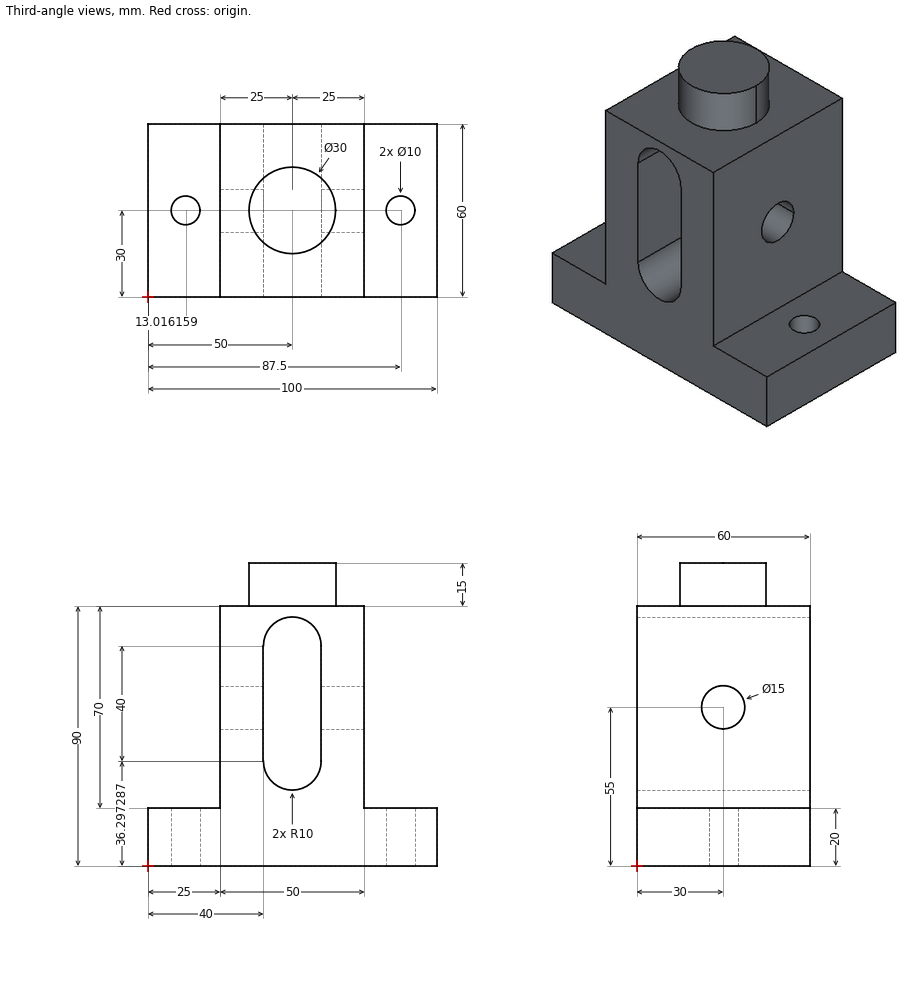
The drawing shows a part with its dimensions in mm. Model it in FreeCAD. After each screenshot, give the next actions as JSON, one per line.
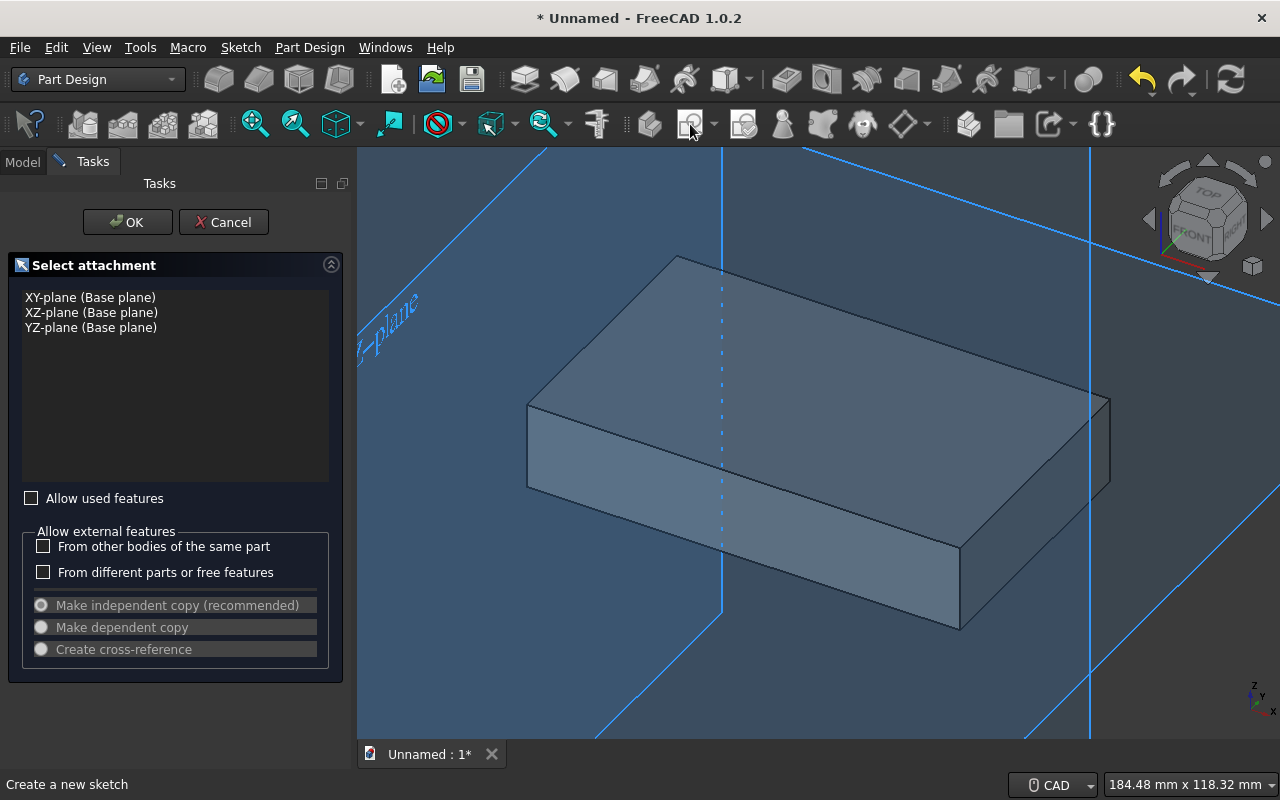
{"action": "left_click", "coordinate": [82, 312]}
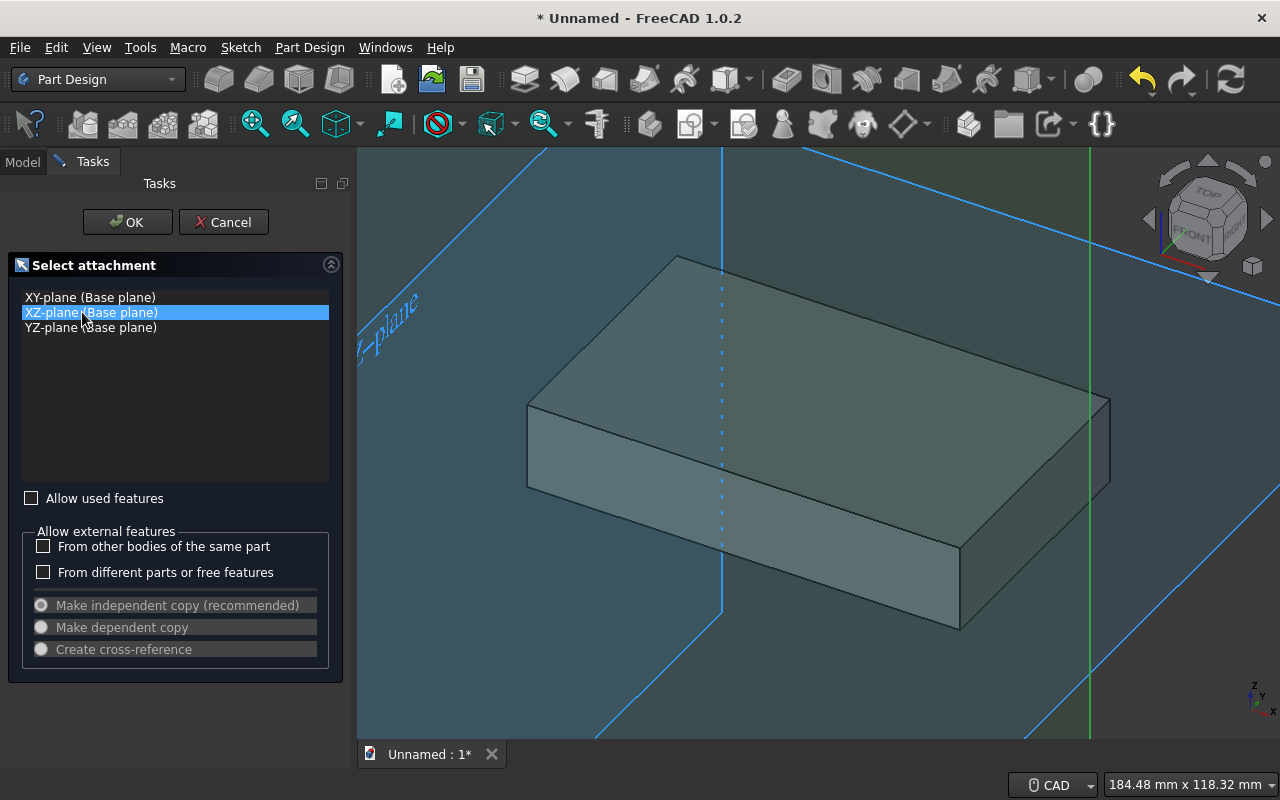
{"action": "left_click", "coordinate": [128, 222]}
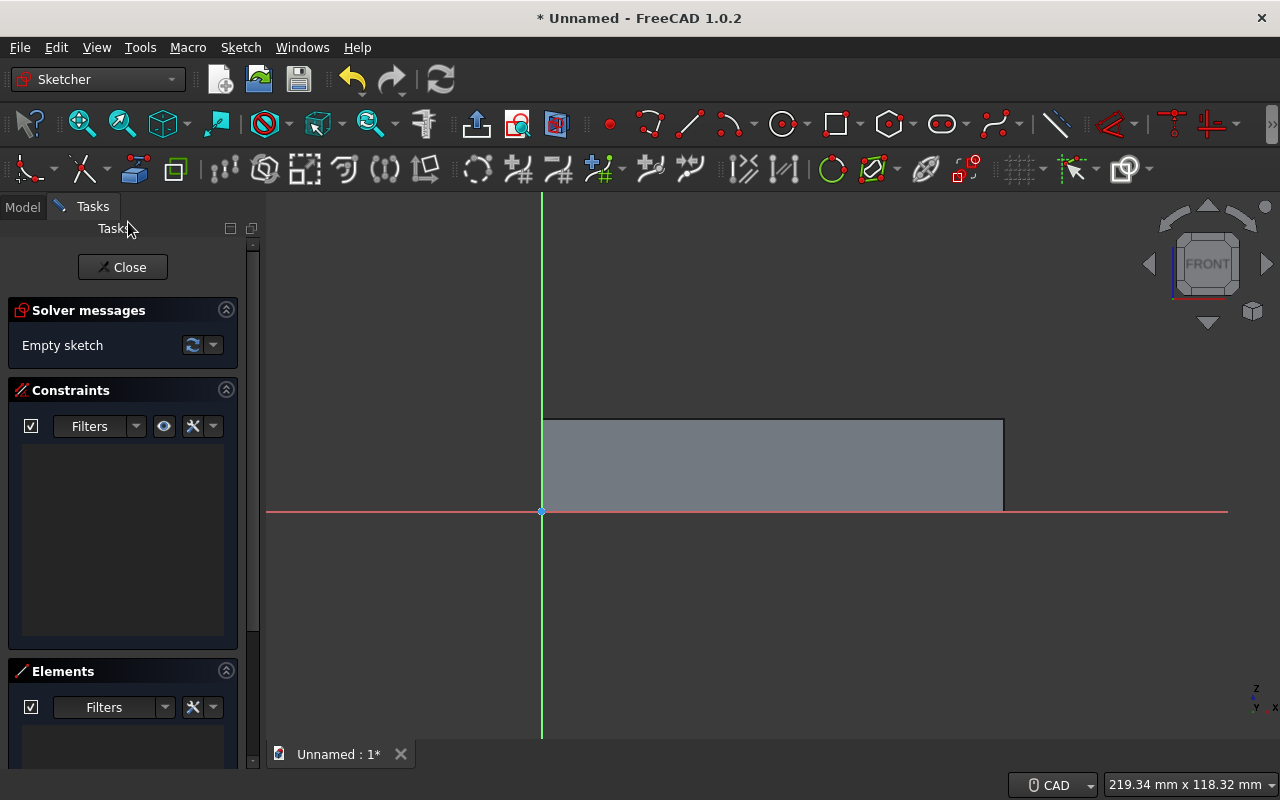
{"action": "scroll", "coordinate": [683, 711], "scroll_direction": "down", "scroll_amount": 2}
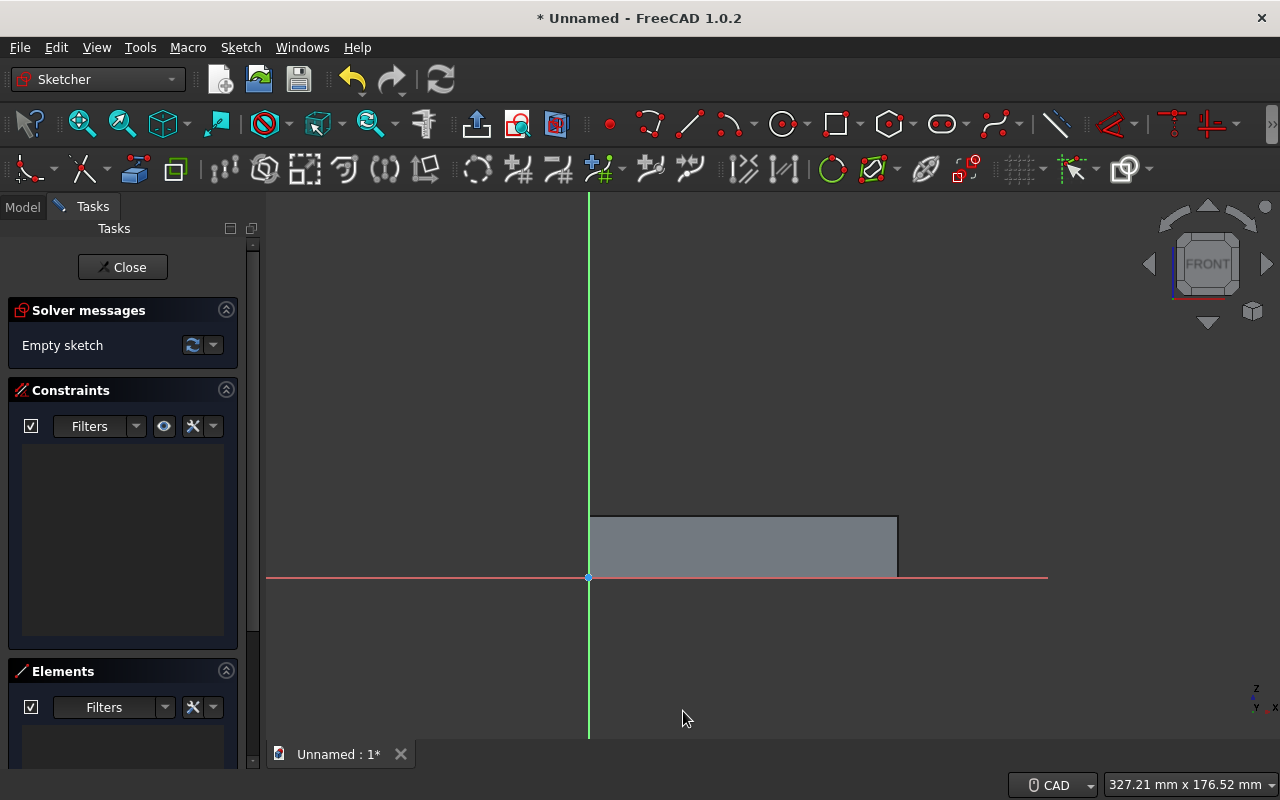
{"action": "key", "text": "g r"}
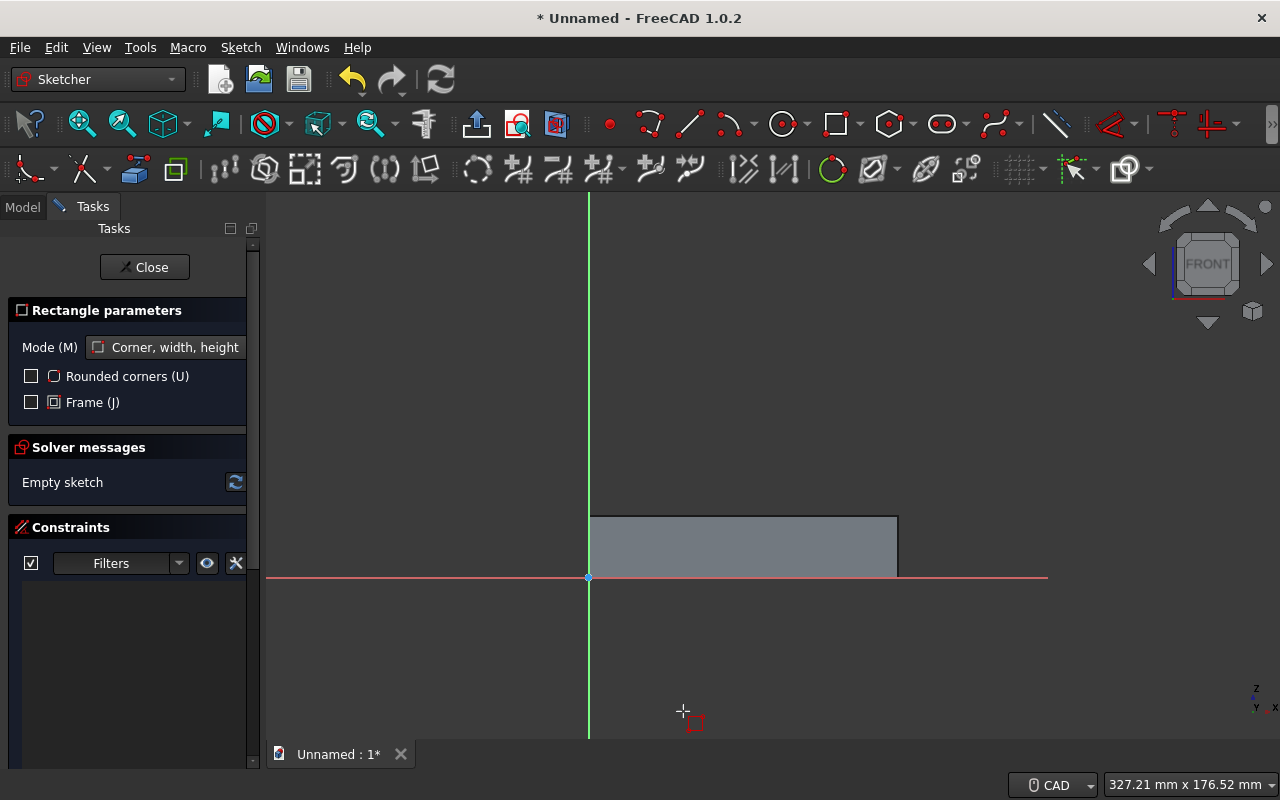
{"action": "left_click", "coordinate": [666, 299]}
{"action": "left_click", "coordinate": [821, 516]}
{"action": "key", "text": "Escape"}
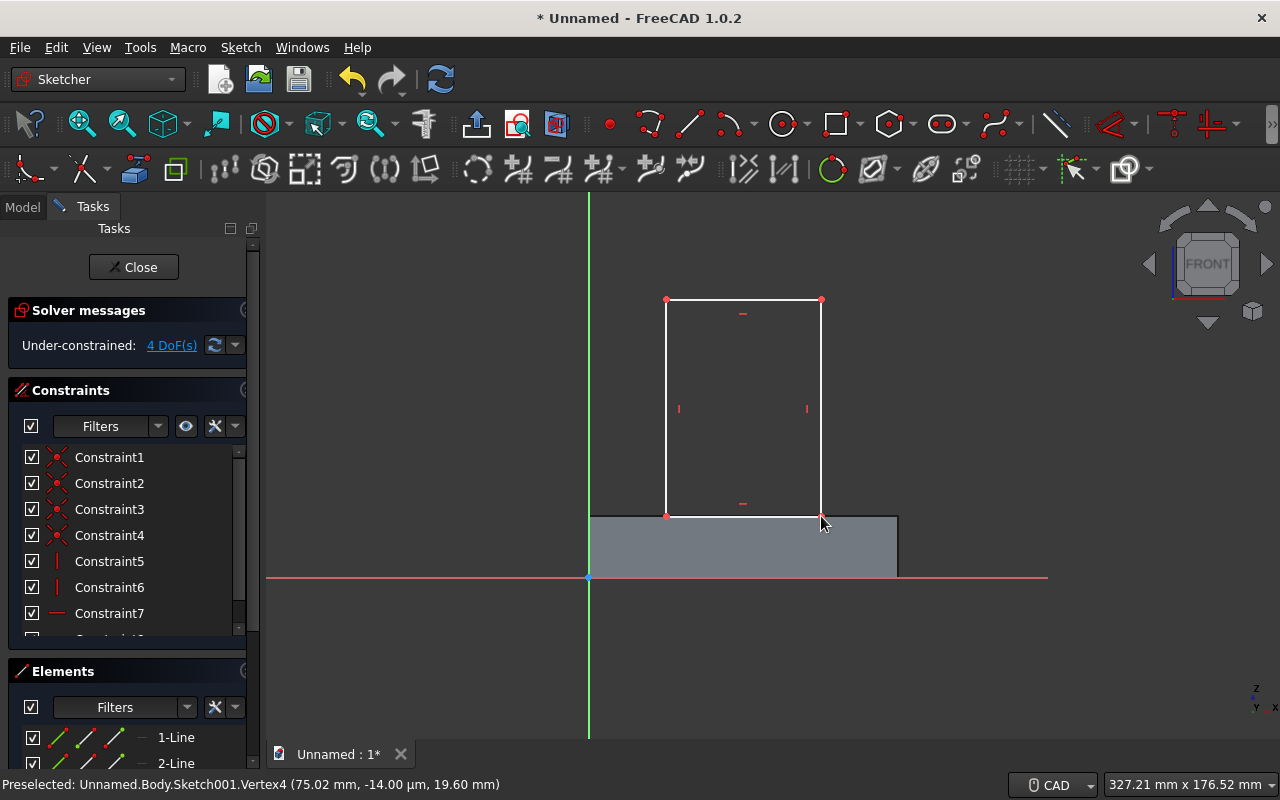
{"action": "left_click", "coordinate": [666, 365]}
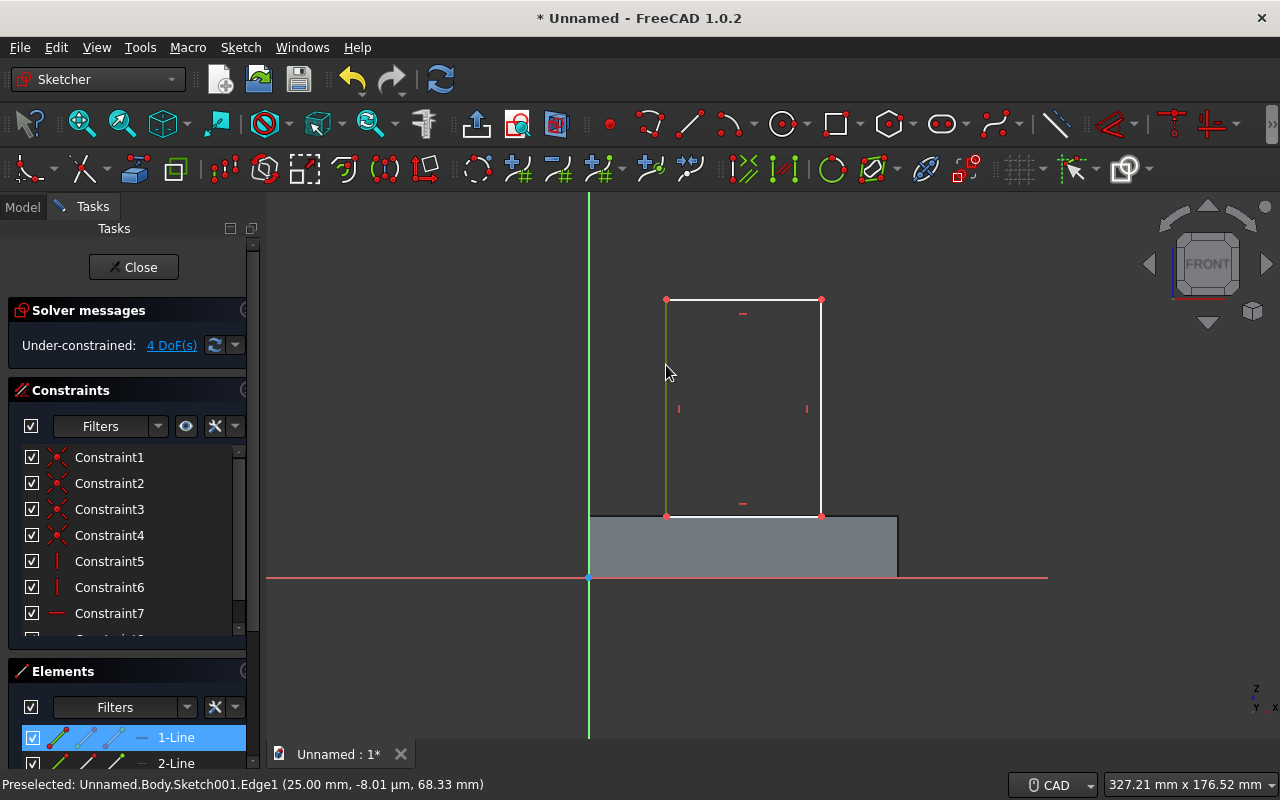
{"action": "key", "text": "i"}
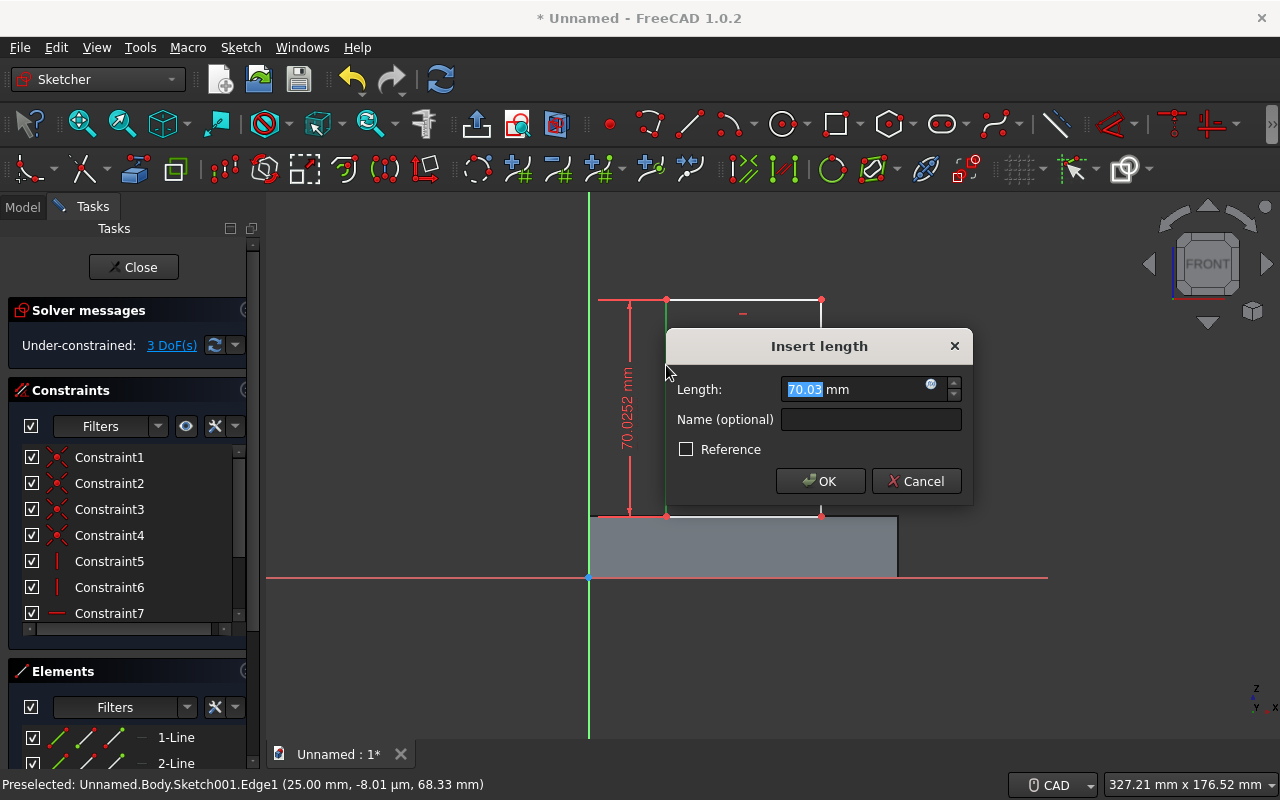
{"action": "type", "text": "70"}
{"action": "key", "text": "Return"}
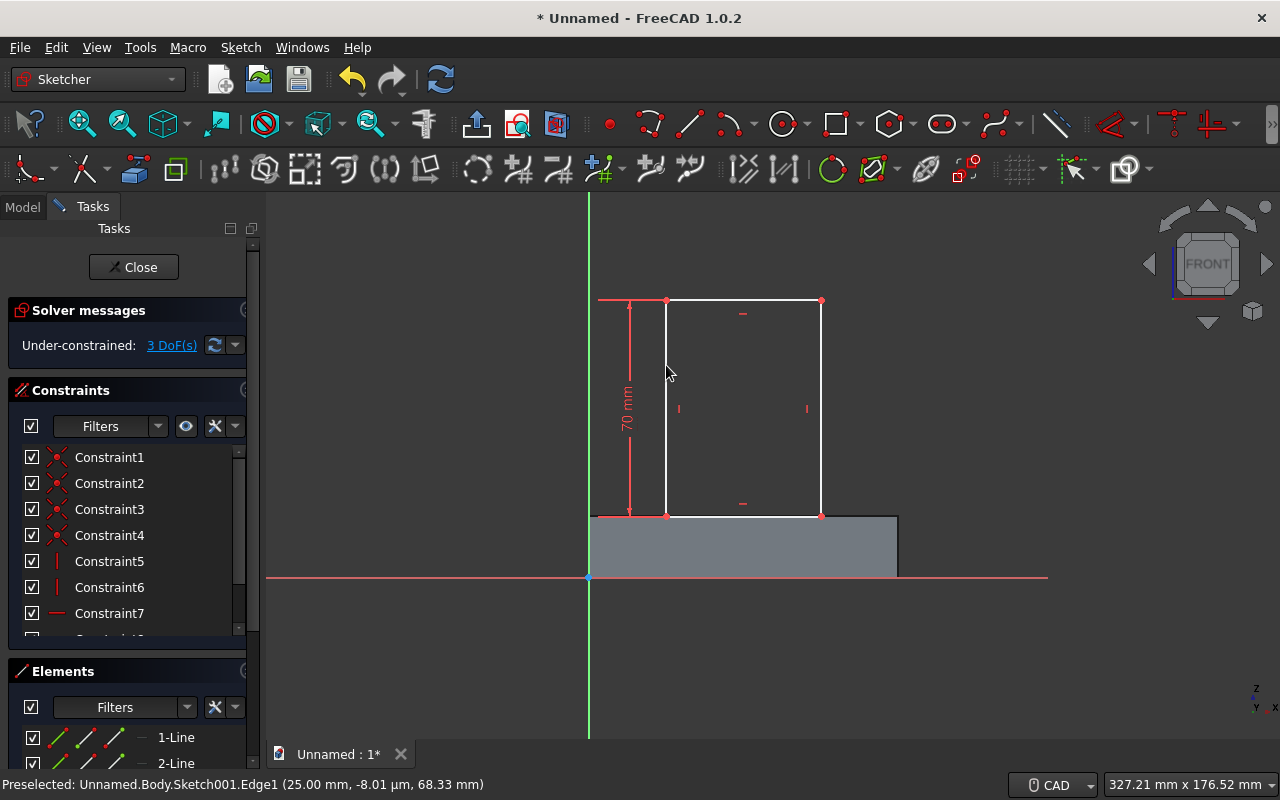
{"action": "left_click", "coordinate": [713, 517]}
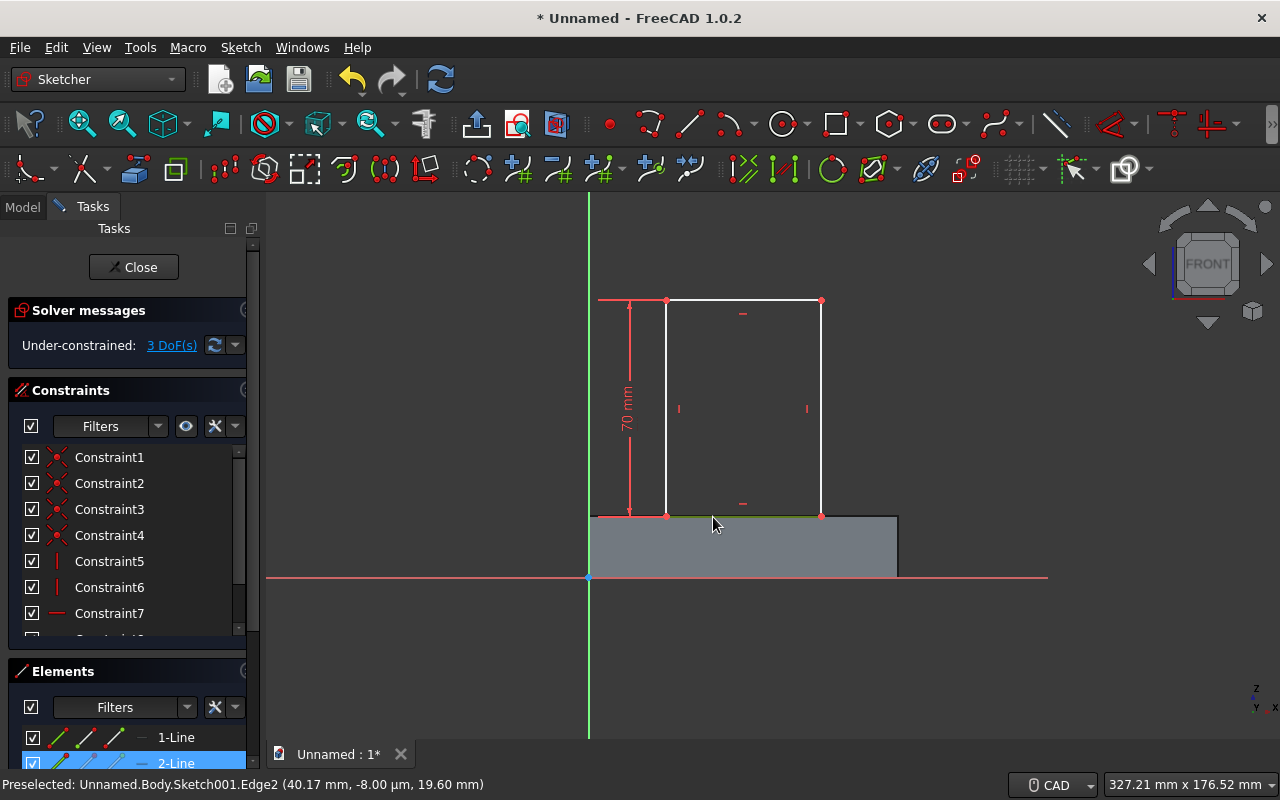
{"action": "key", "text": "l"}